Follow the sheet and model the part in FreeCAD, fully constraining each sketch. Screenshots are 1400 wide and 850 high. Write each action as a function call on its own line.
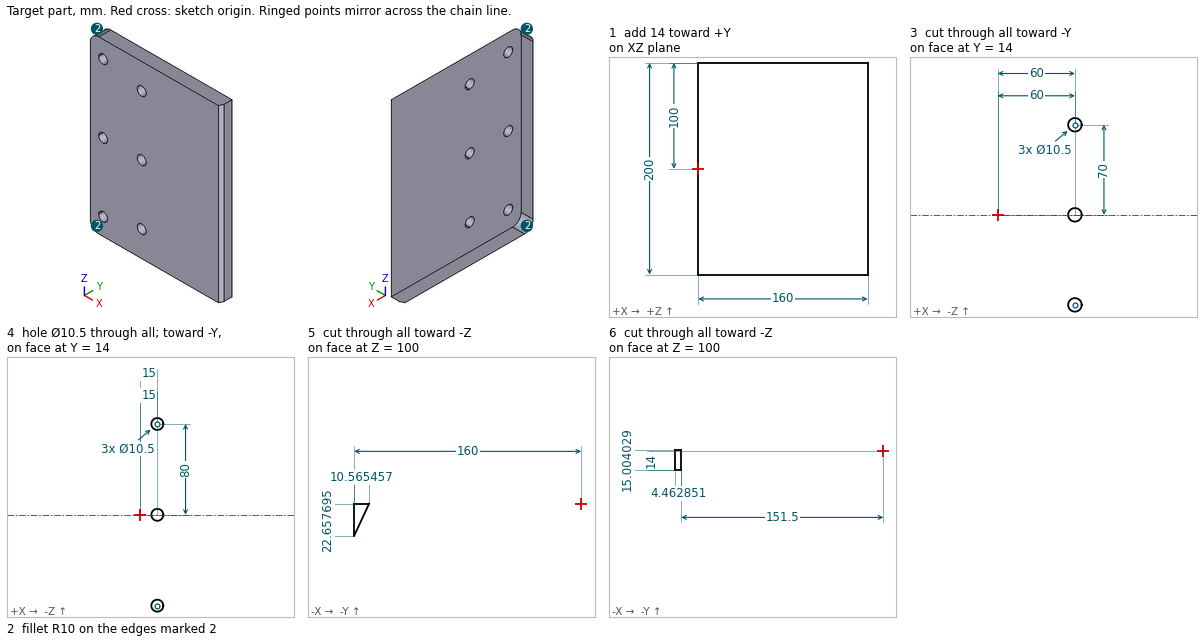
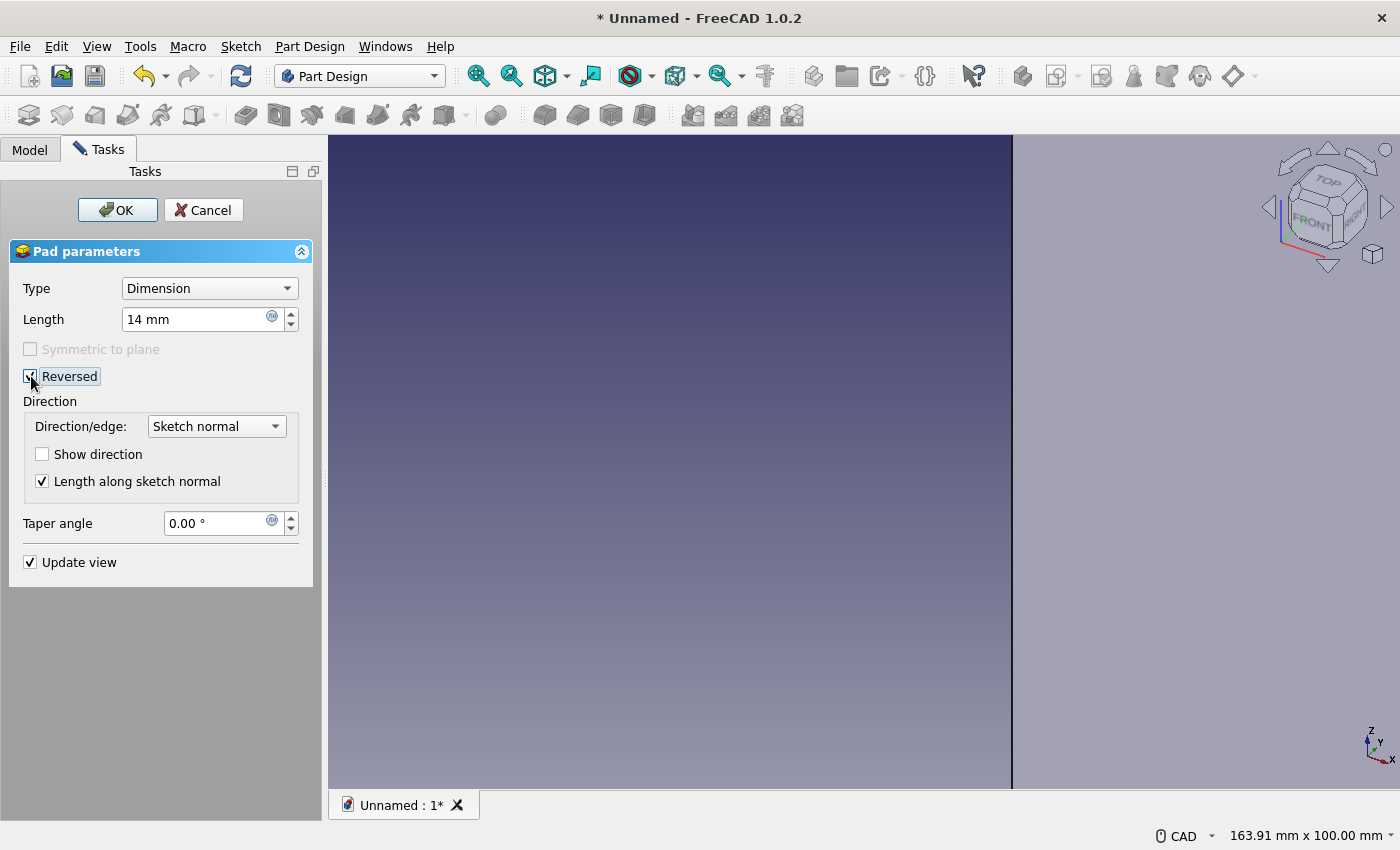
click(118, 210)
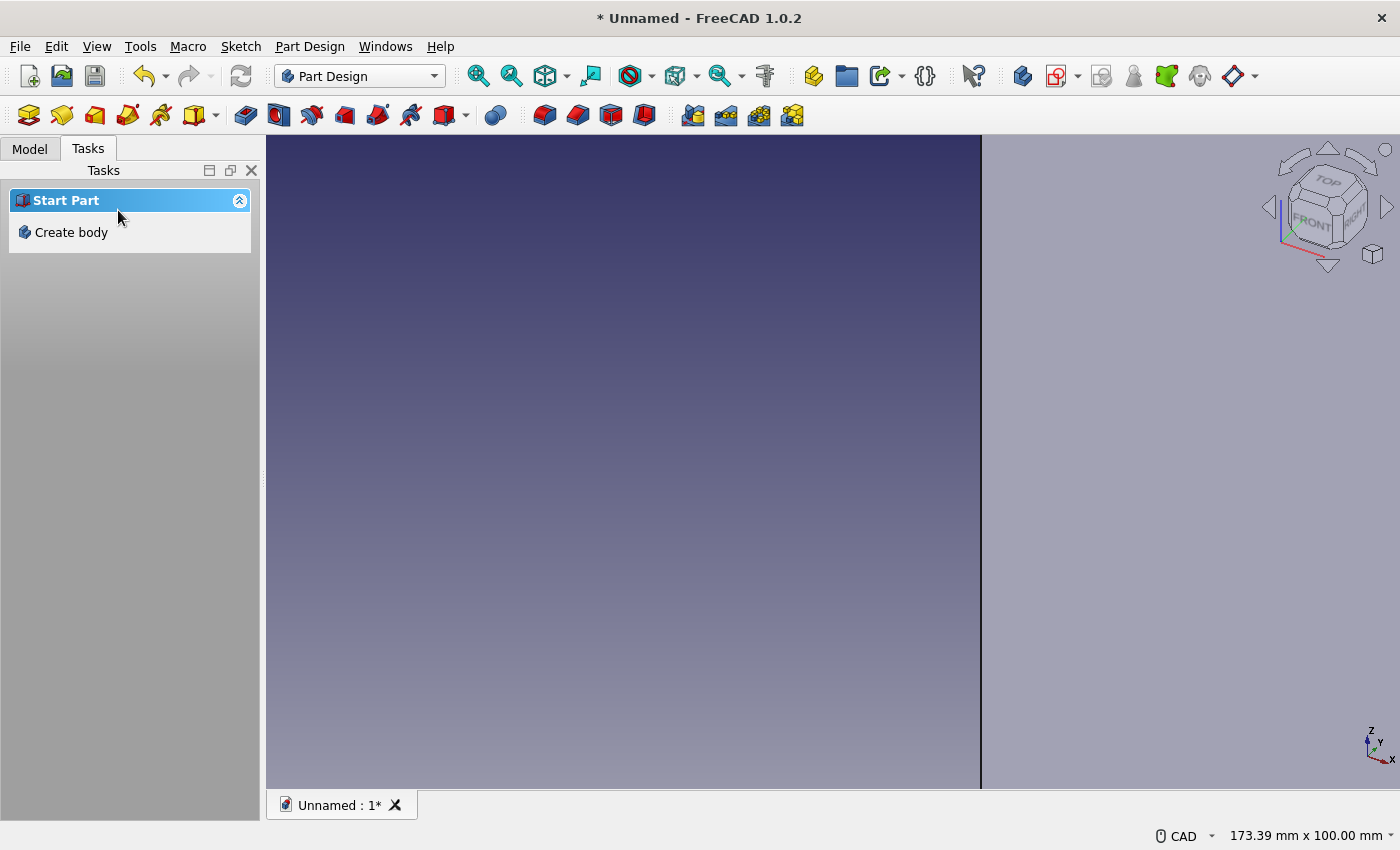
key(v)
key(f)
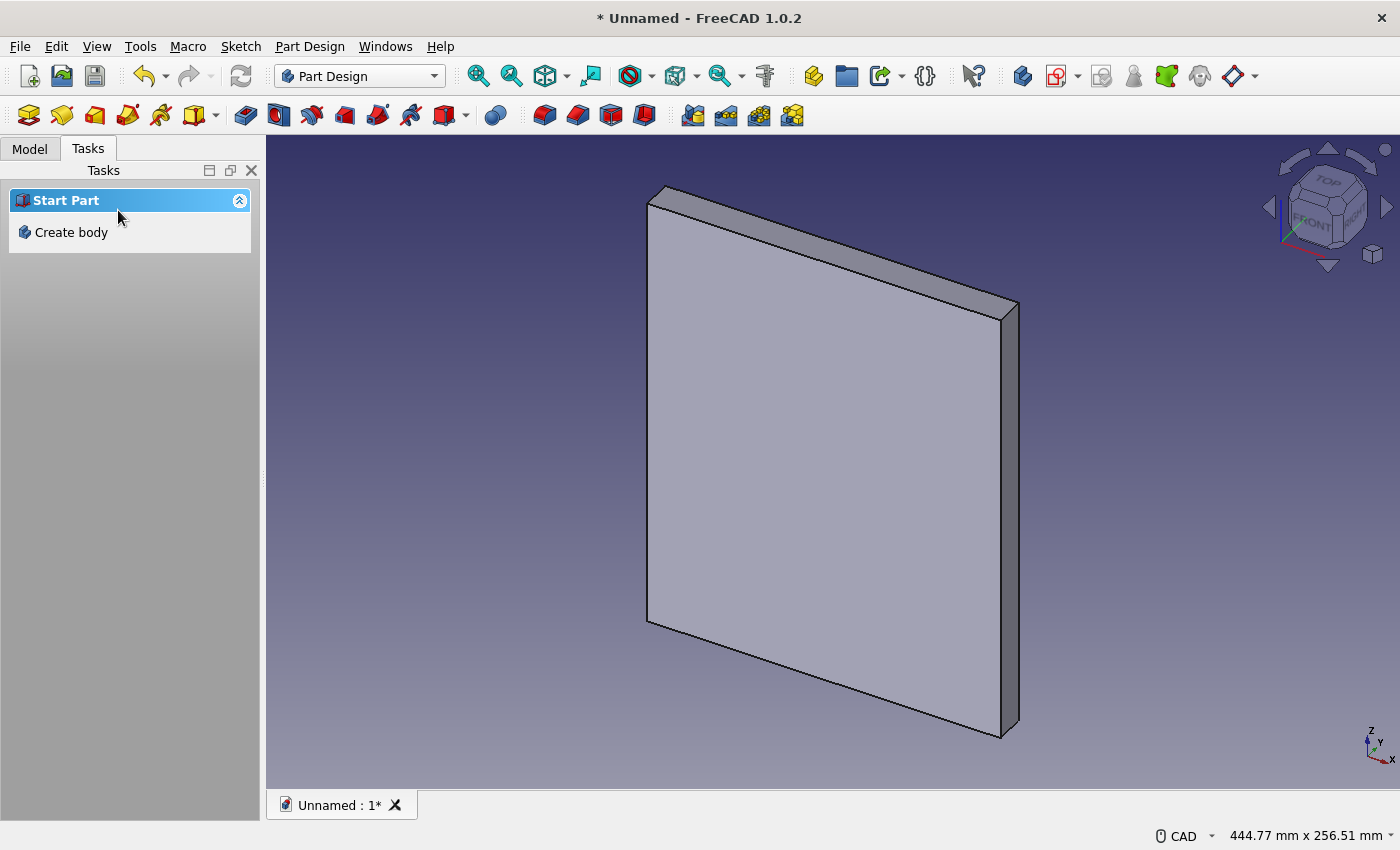
key(0)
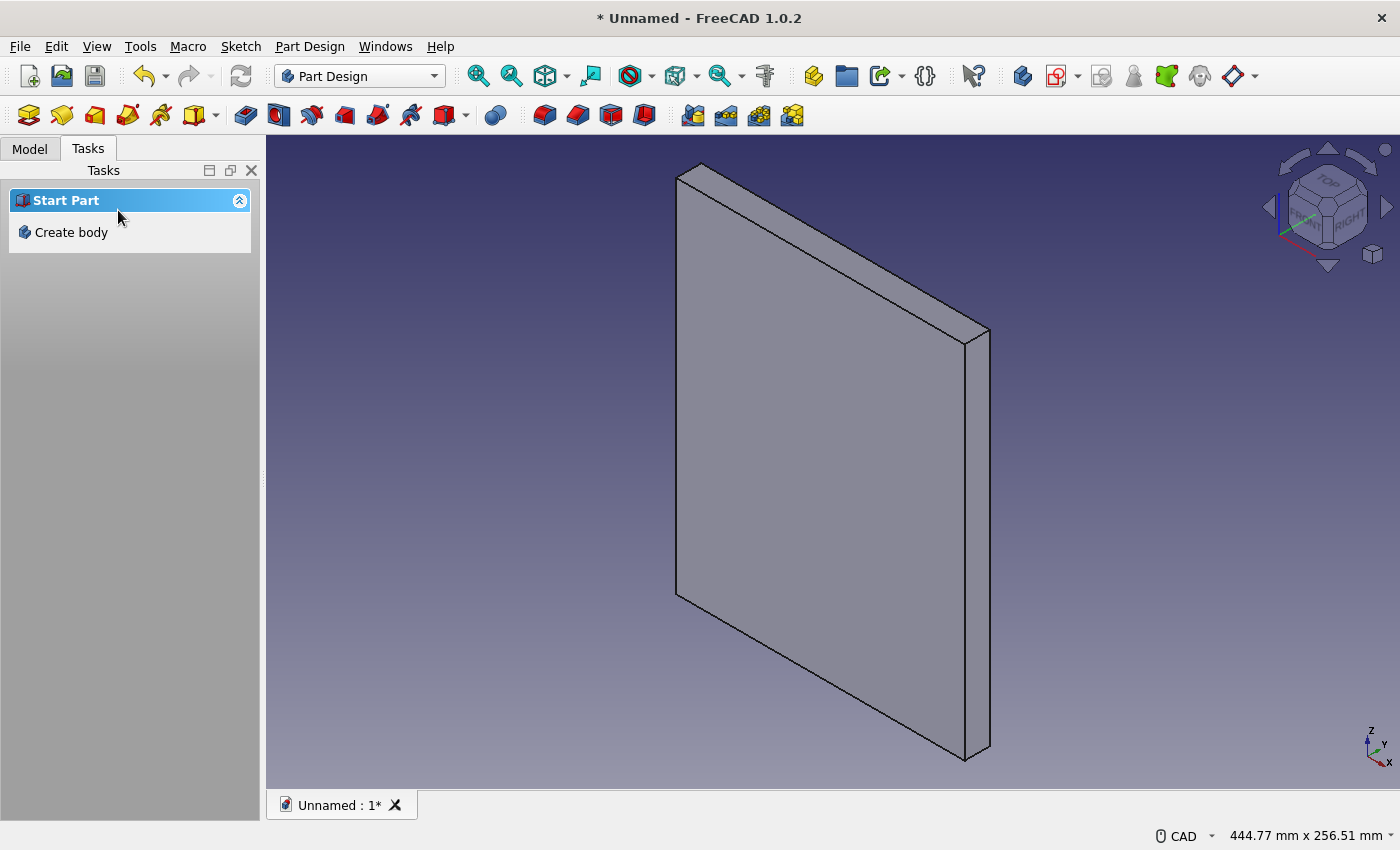
key(2)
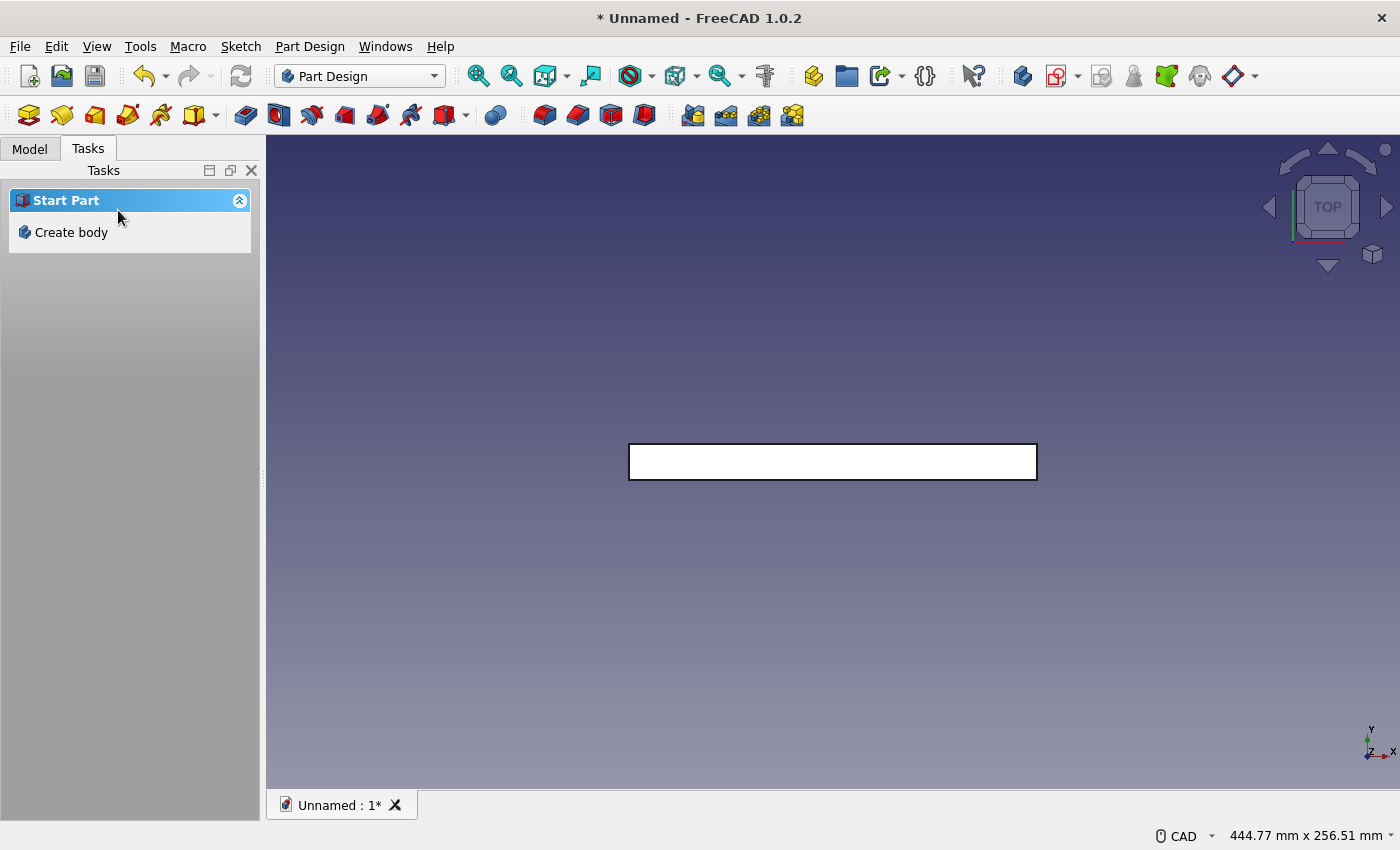
click(479, 76)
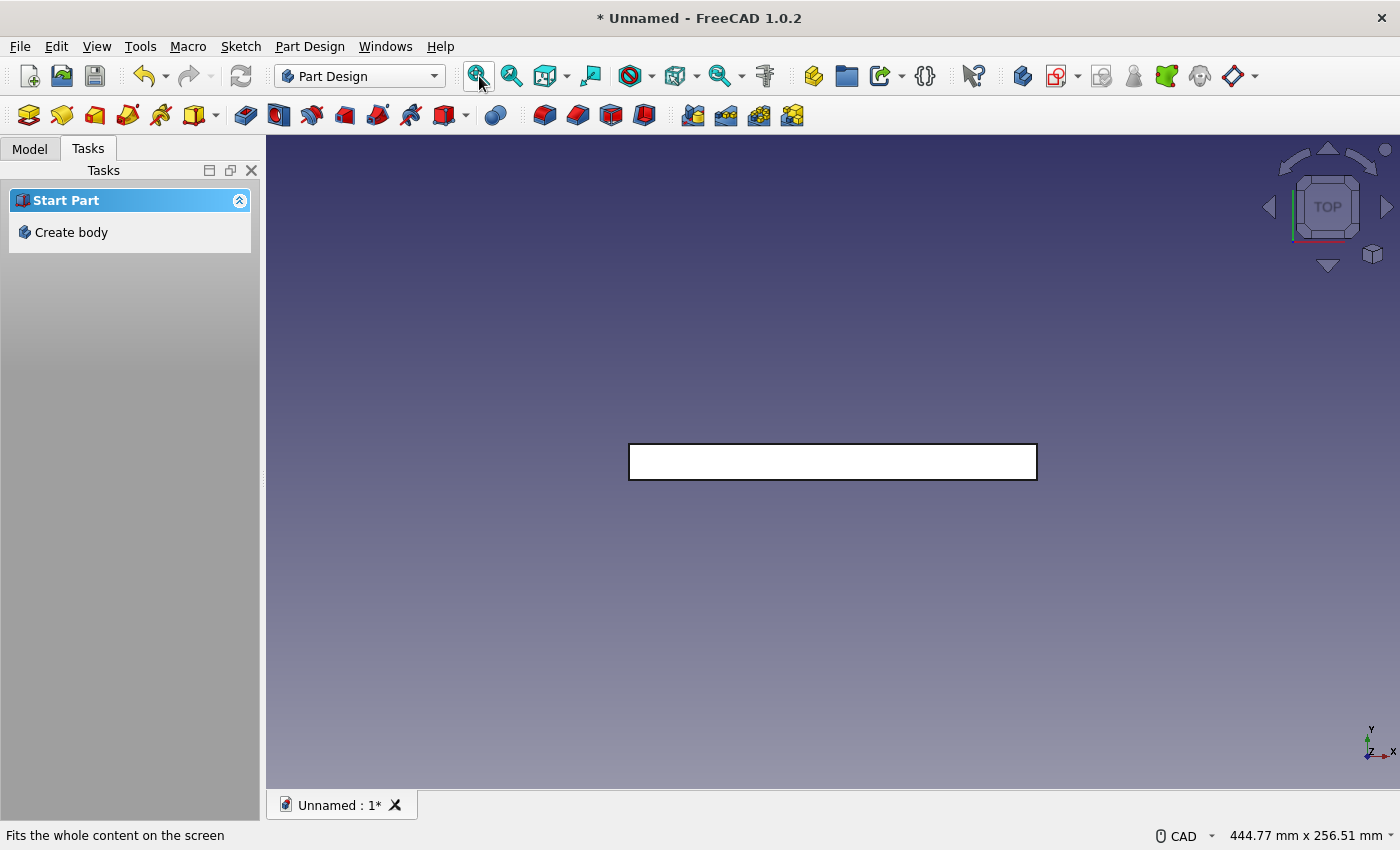
click(629, 461)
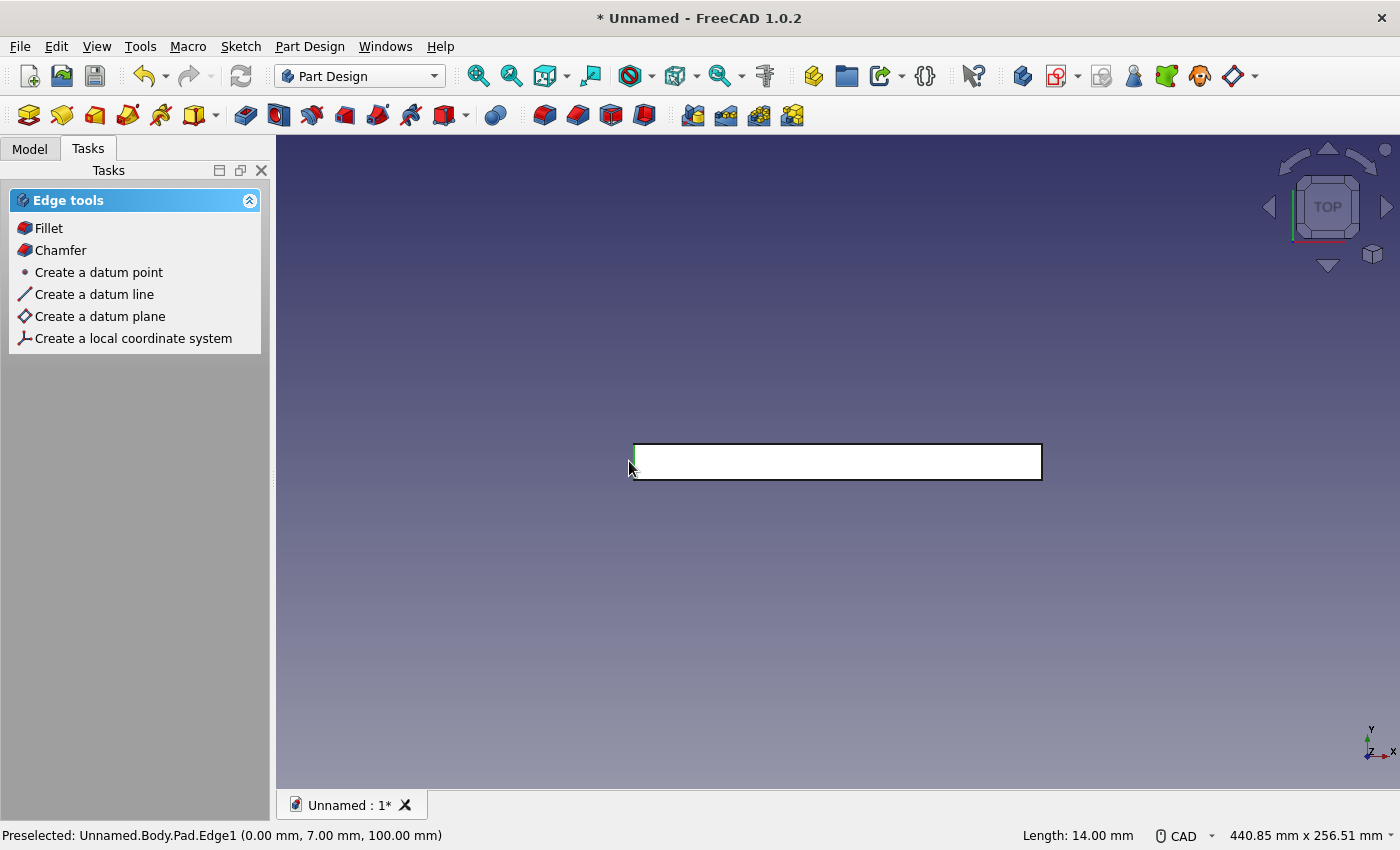
key(1)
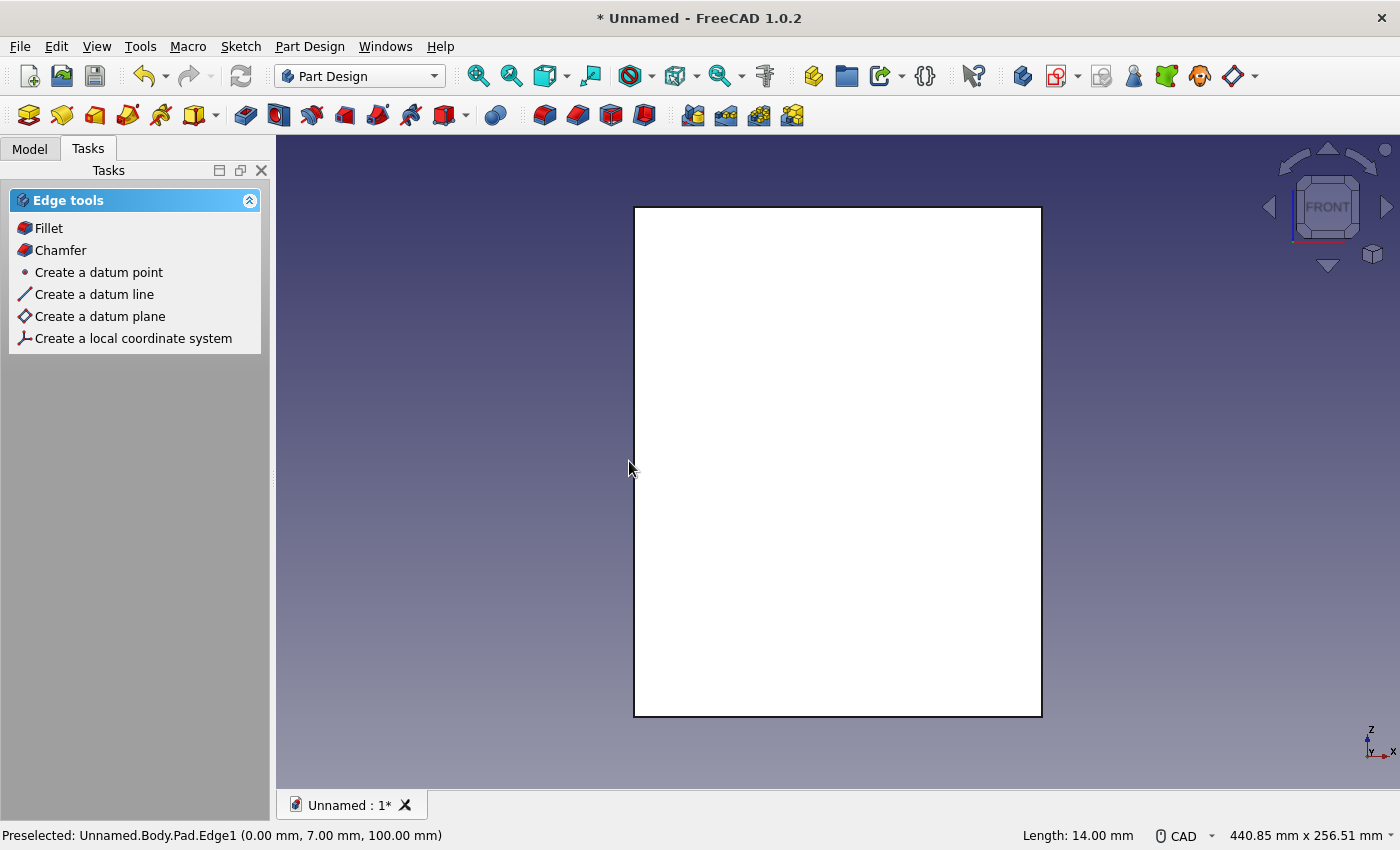
key(3)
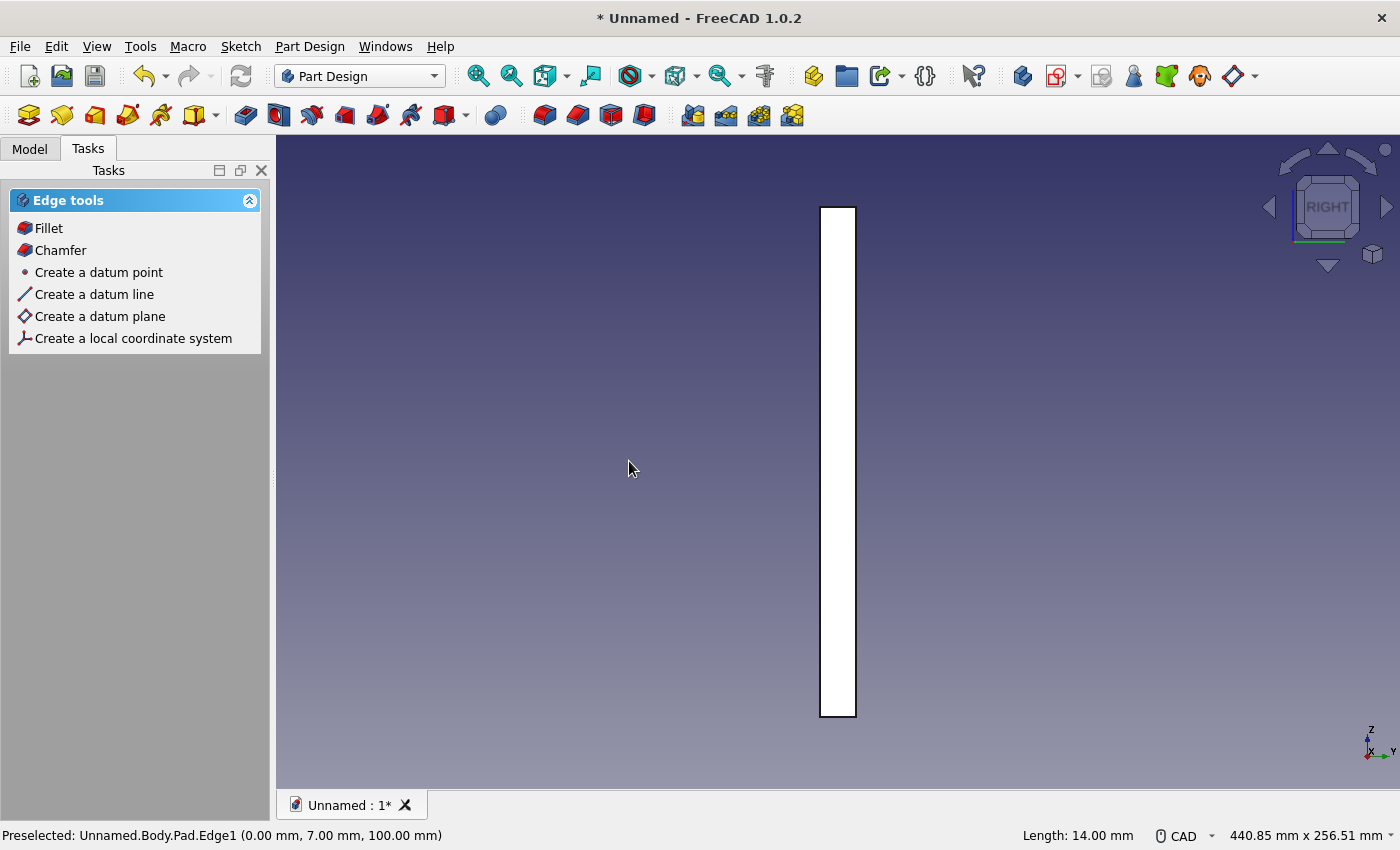
key(5)